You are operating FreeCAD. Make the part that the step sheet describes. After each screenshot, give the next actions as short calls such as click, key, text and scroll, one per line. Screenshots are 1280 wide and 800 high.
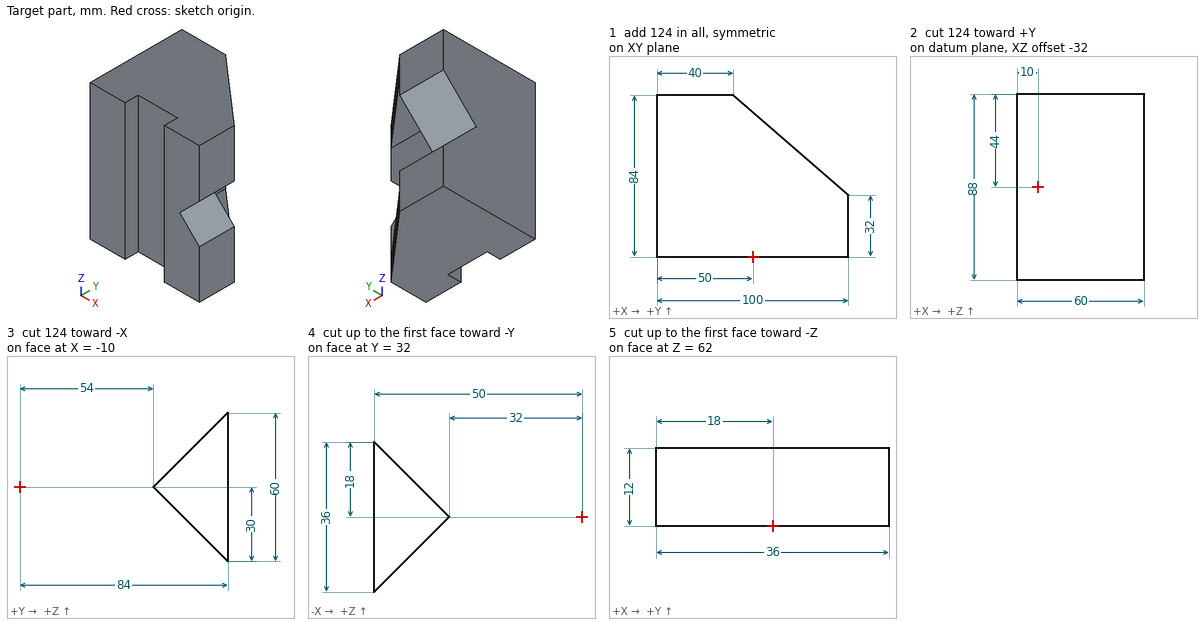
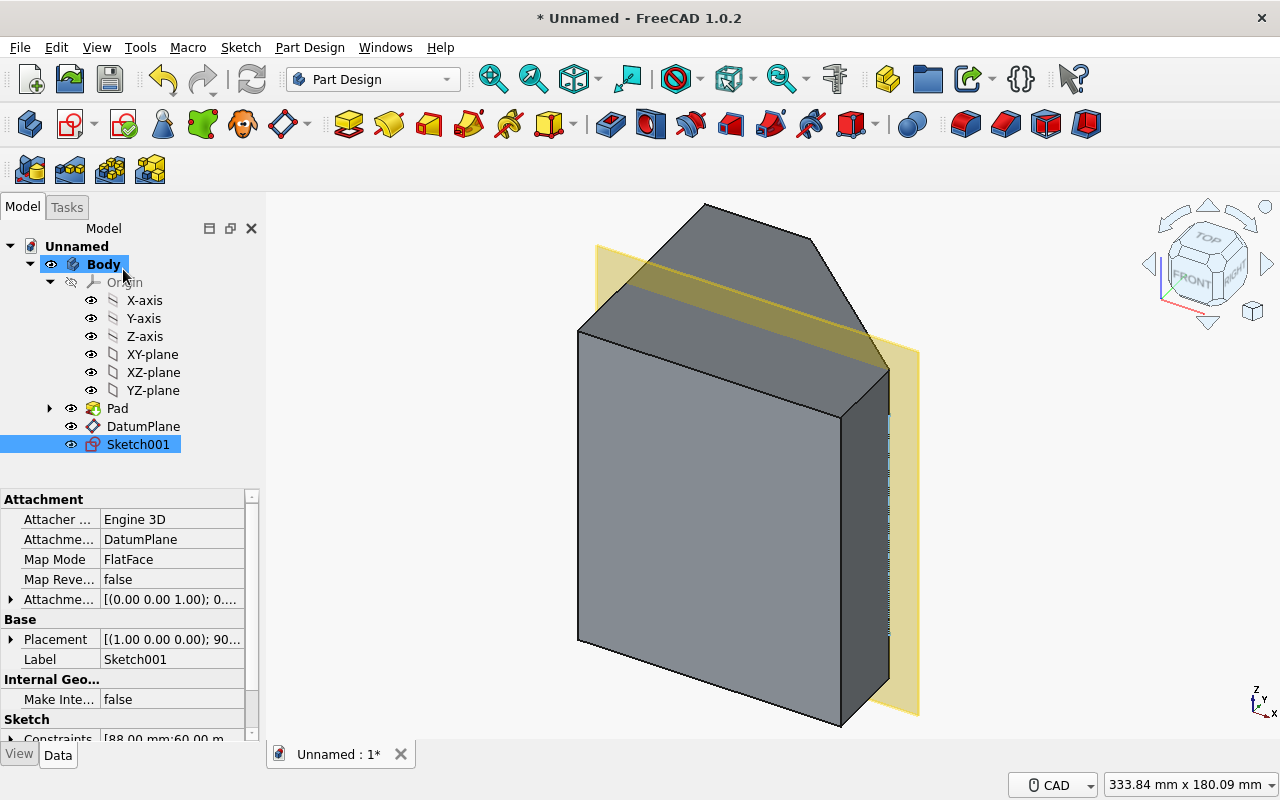
click(612, 124)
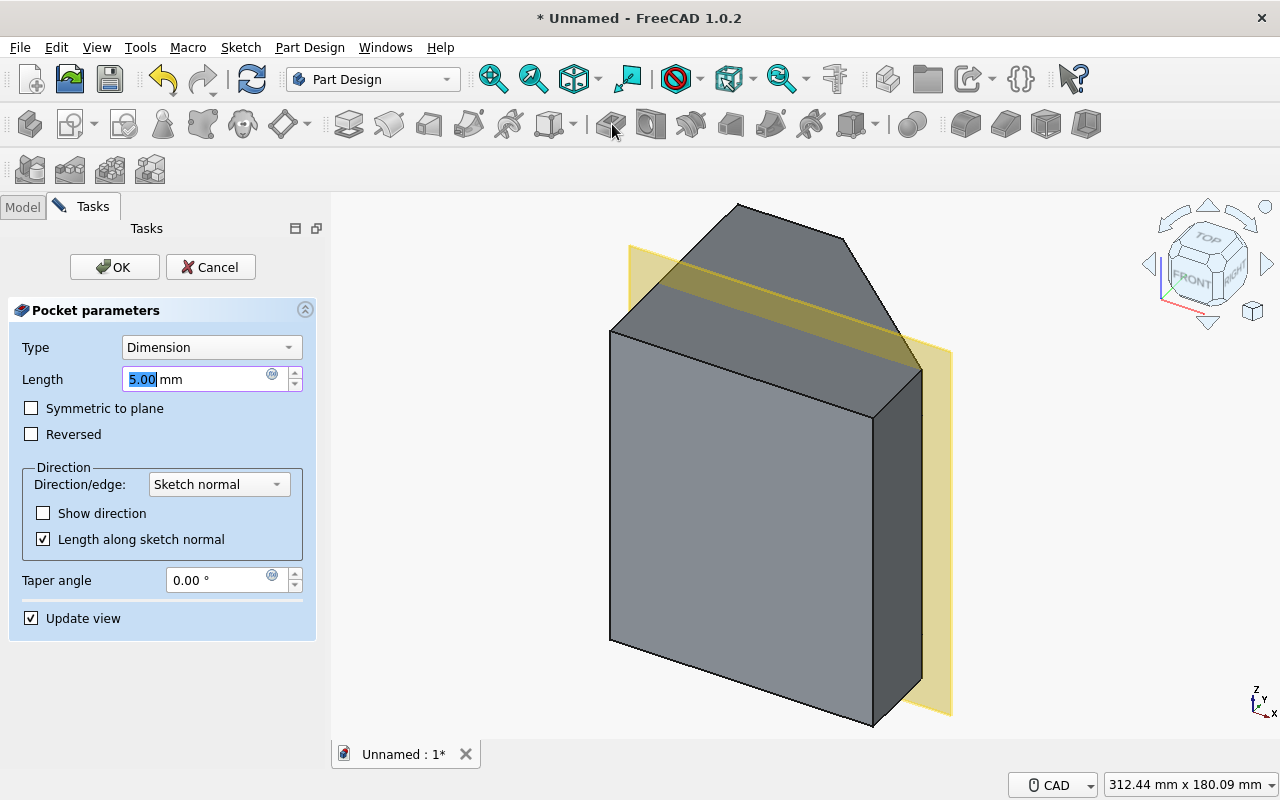
text(124)
key(Tab)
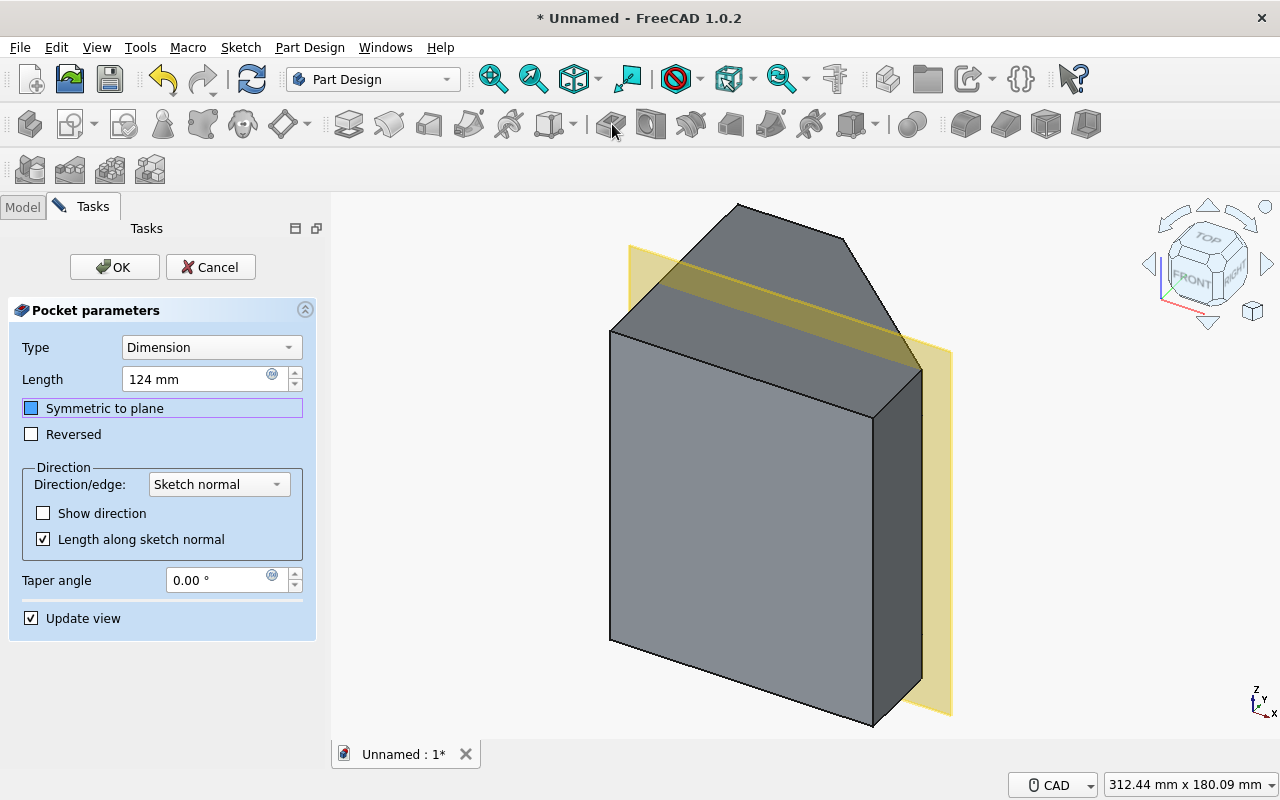
click(115, 267)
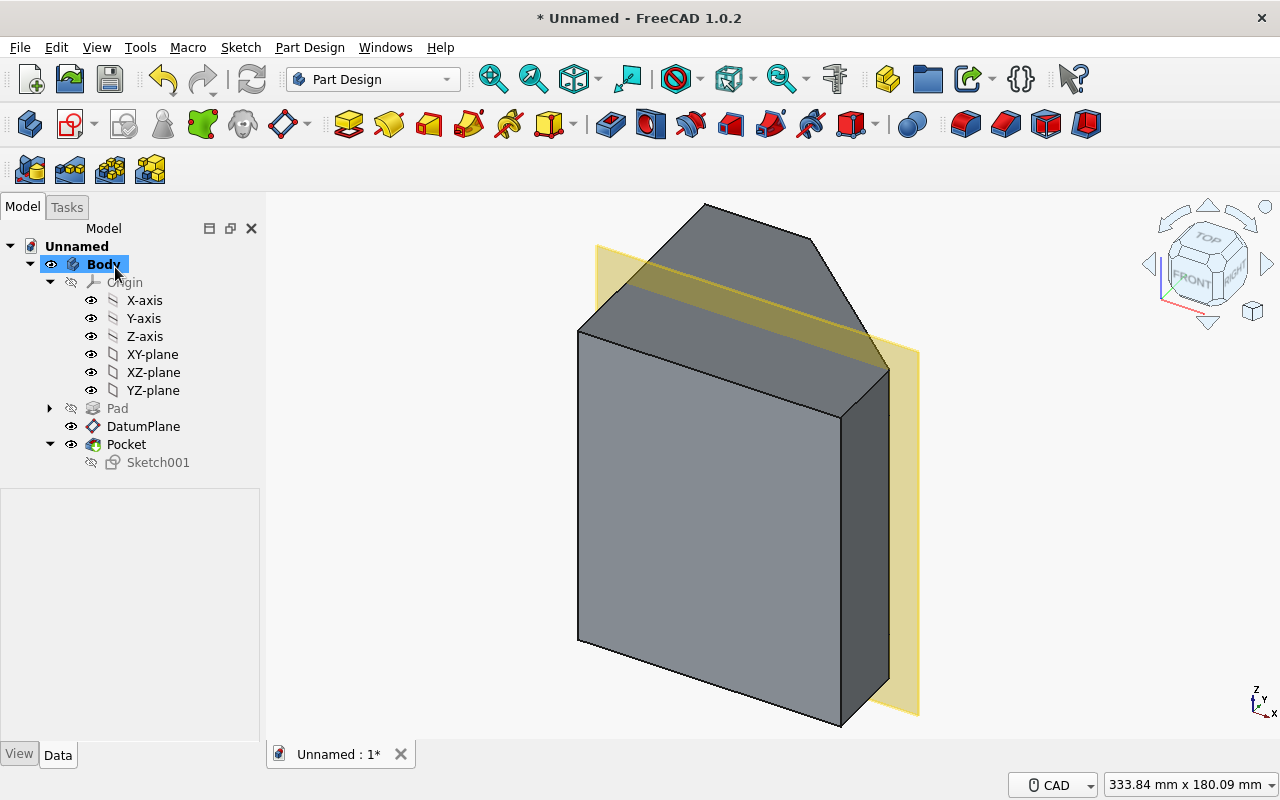
click(116, 426)
key(space)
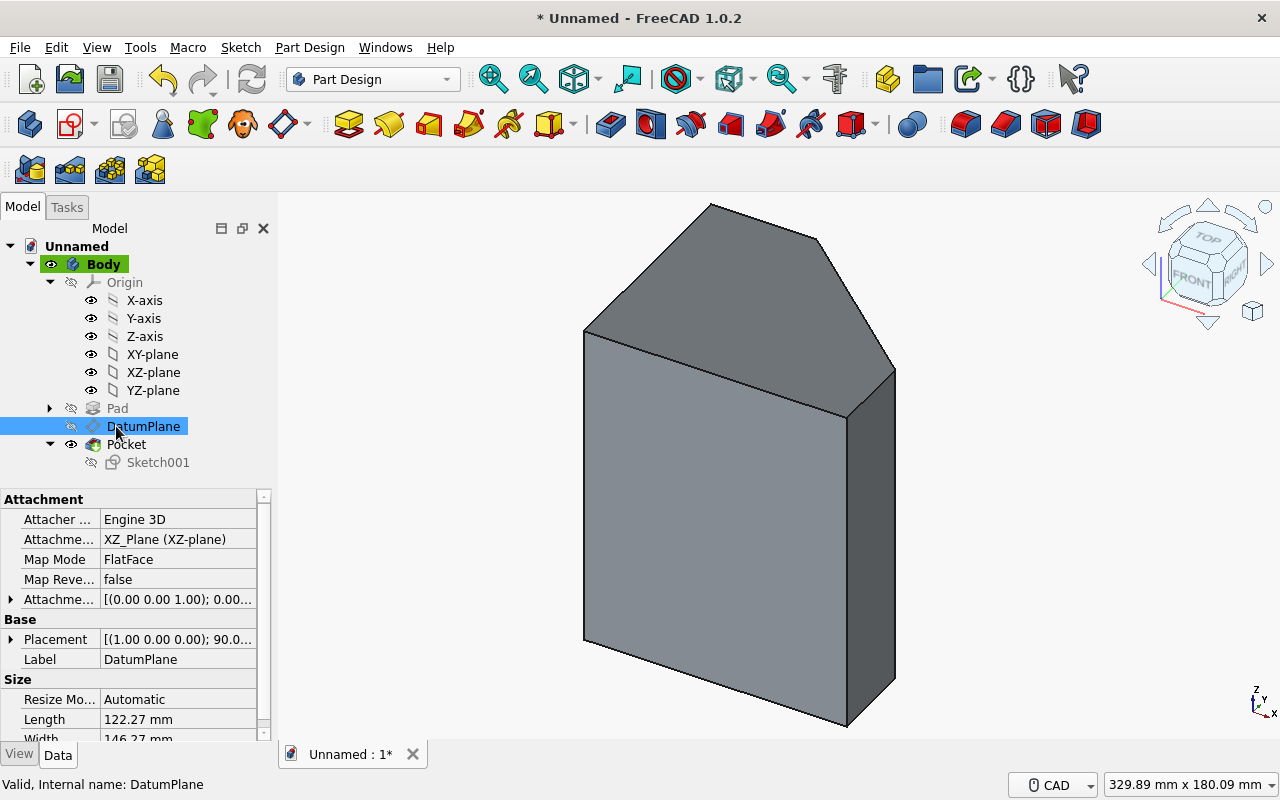
key(0)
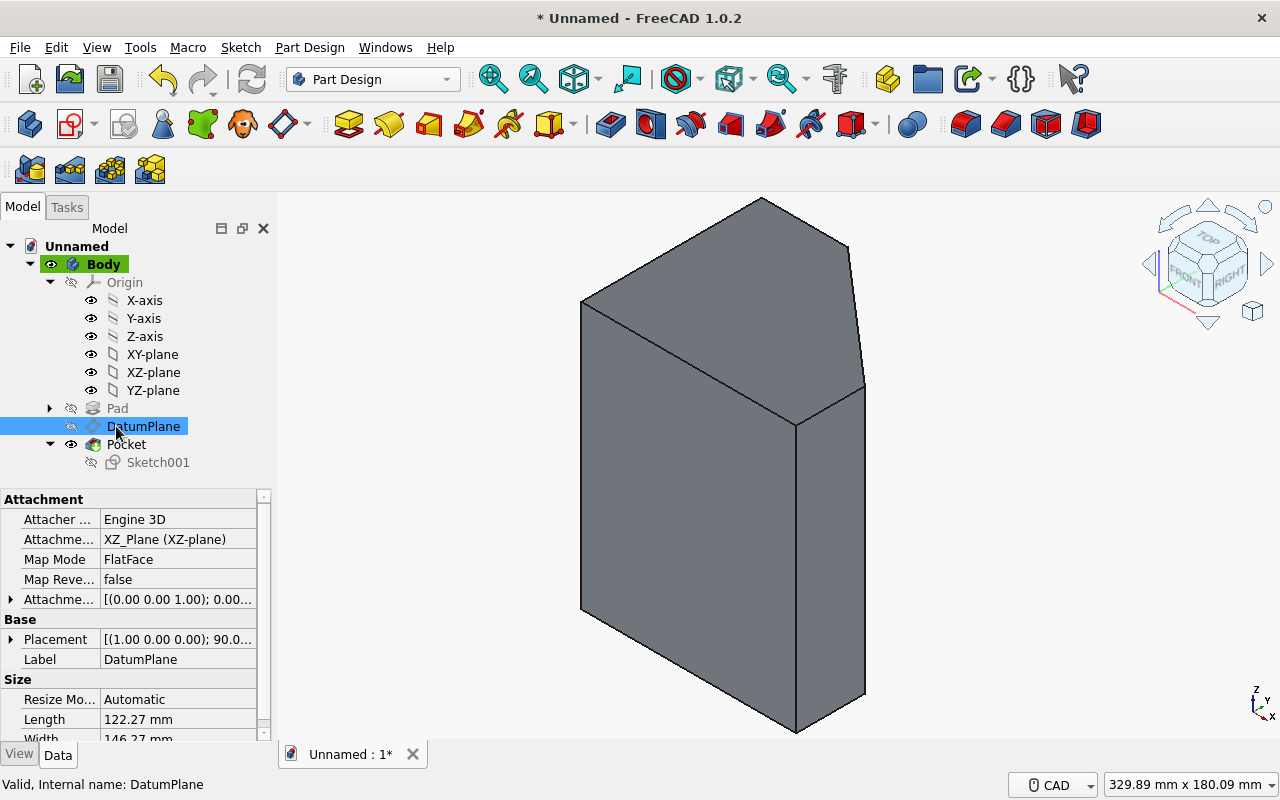
key(3)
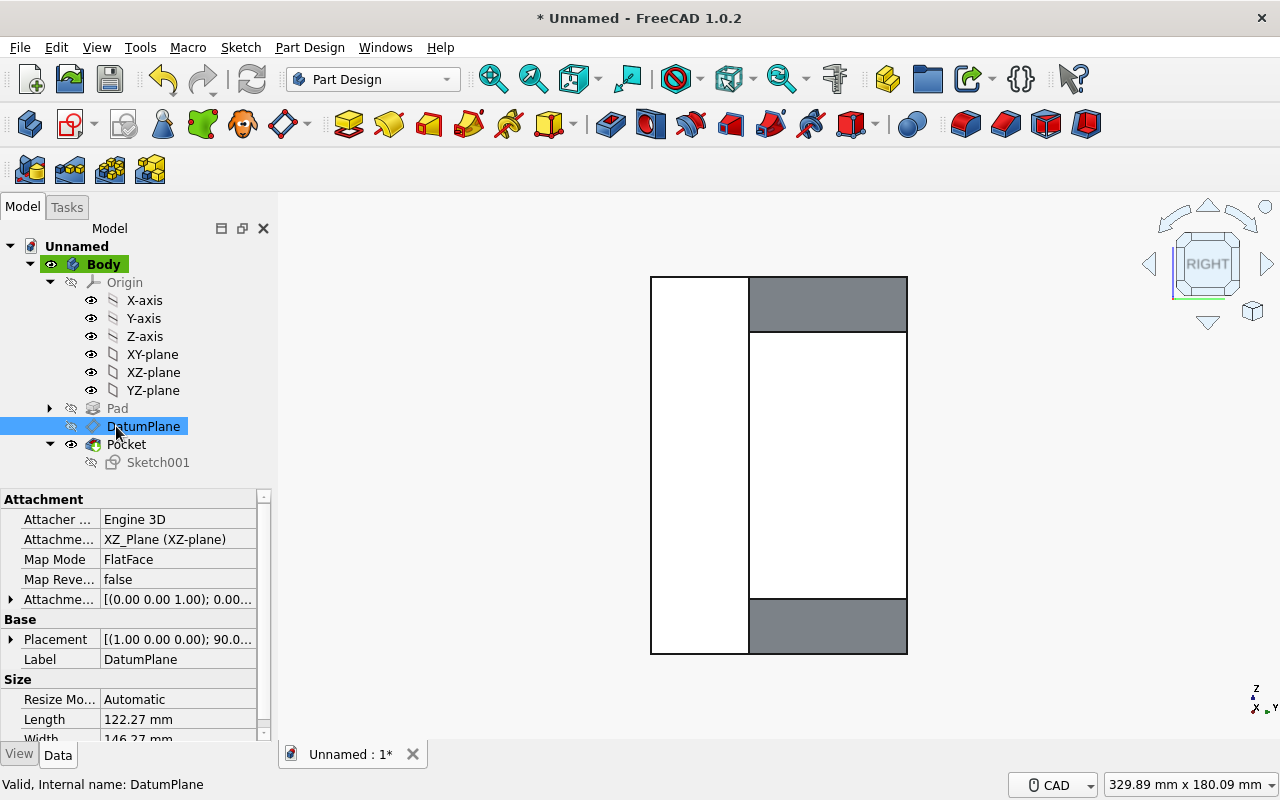
click(828, 464)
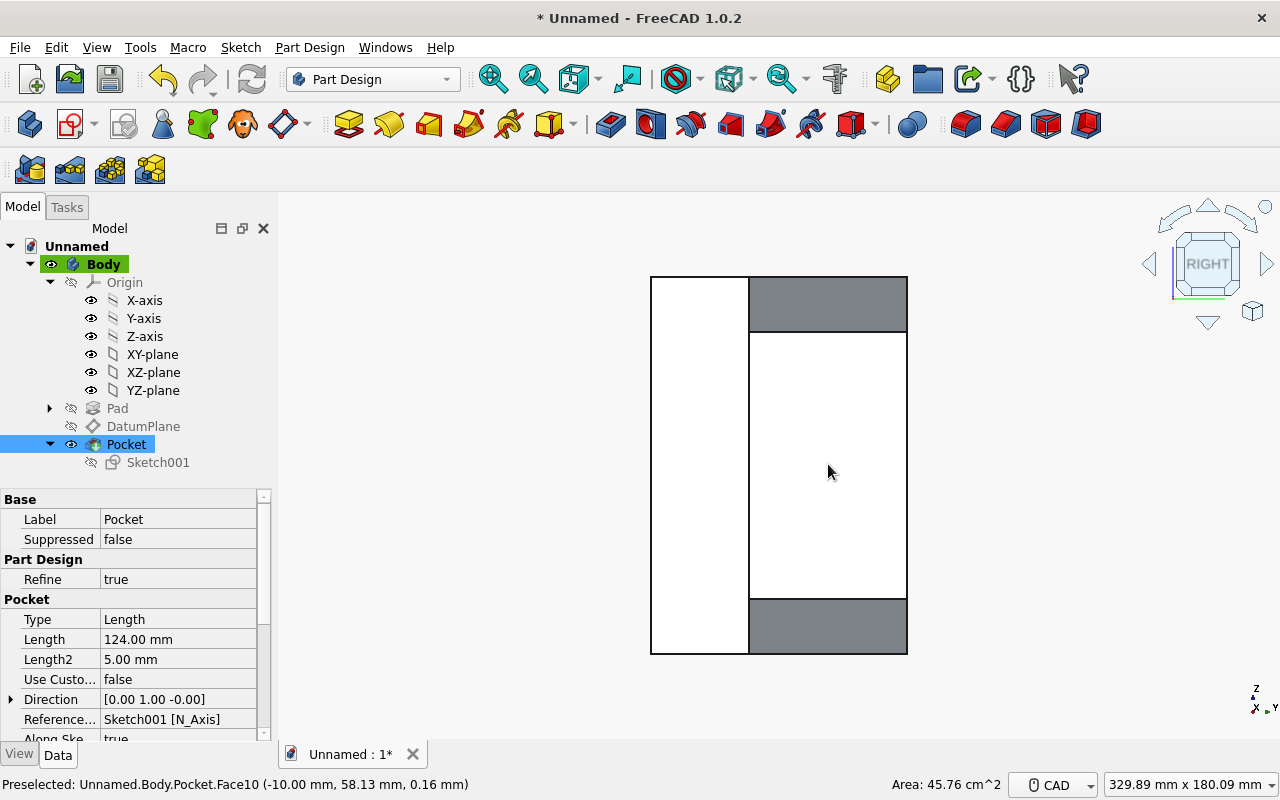
click(70, 124)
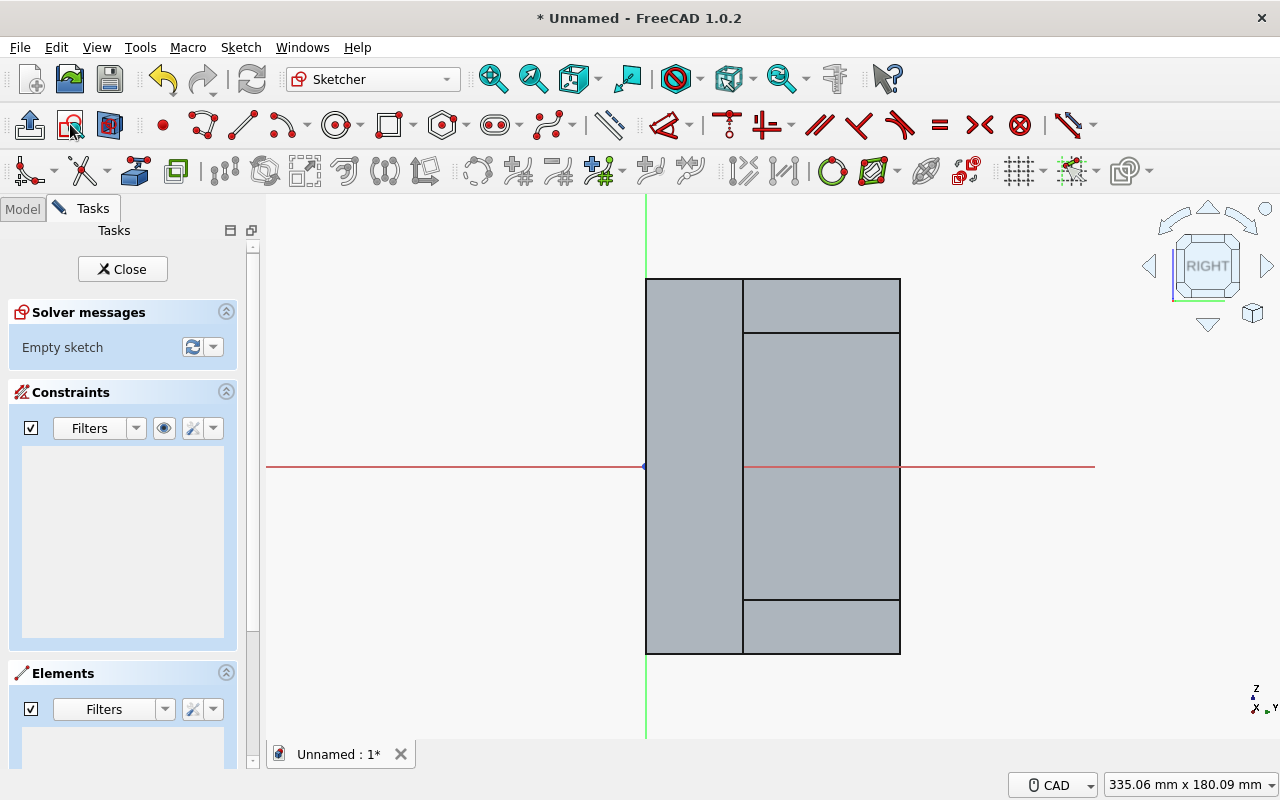
click(110, 126)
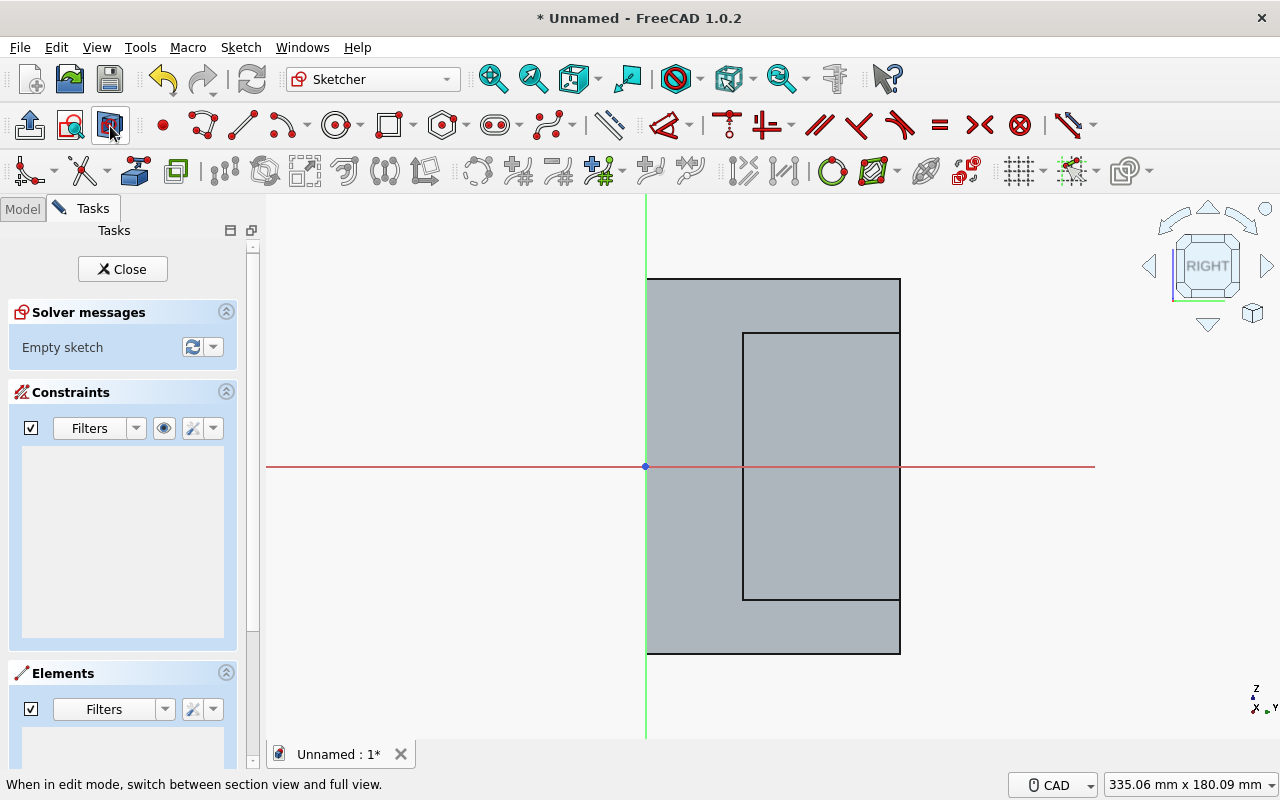
scroll(856, 466, up, 3)